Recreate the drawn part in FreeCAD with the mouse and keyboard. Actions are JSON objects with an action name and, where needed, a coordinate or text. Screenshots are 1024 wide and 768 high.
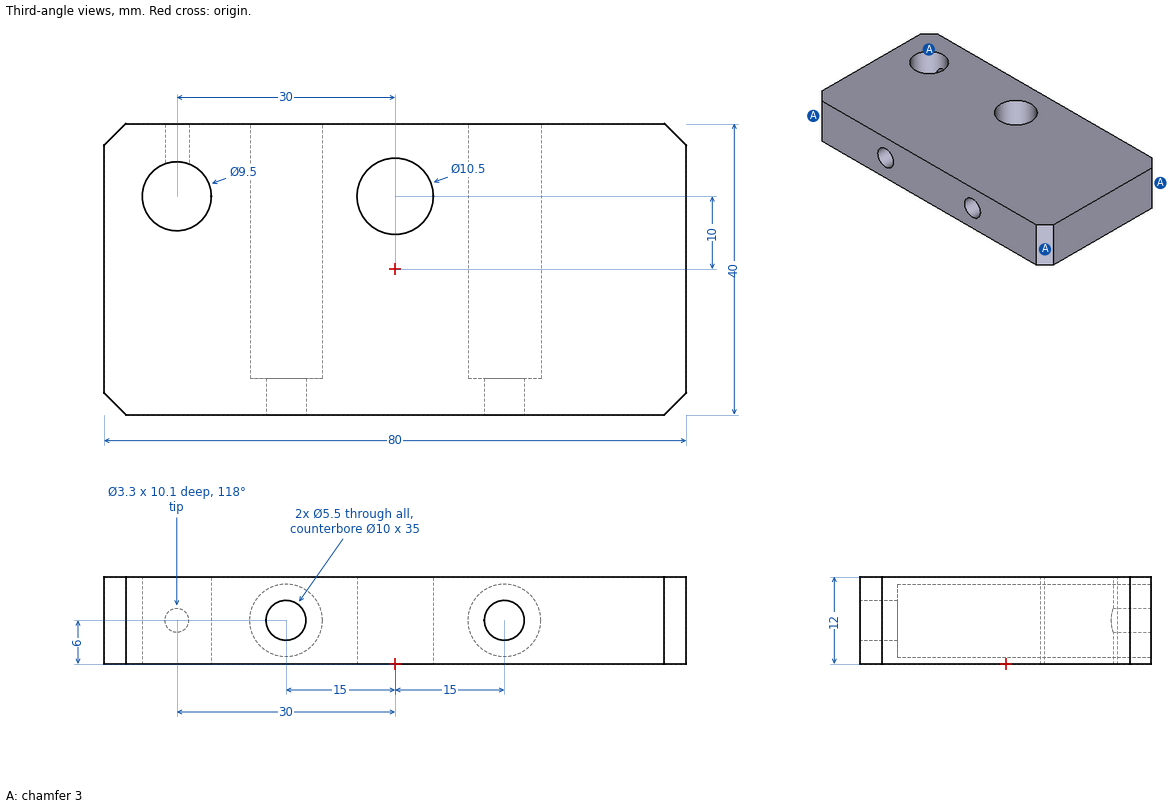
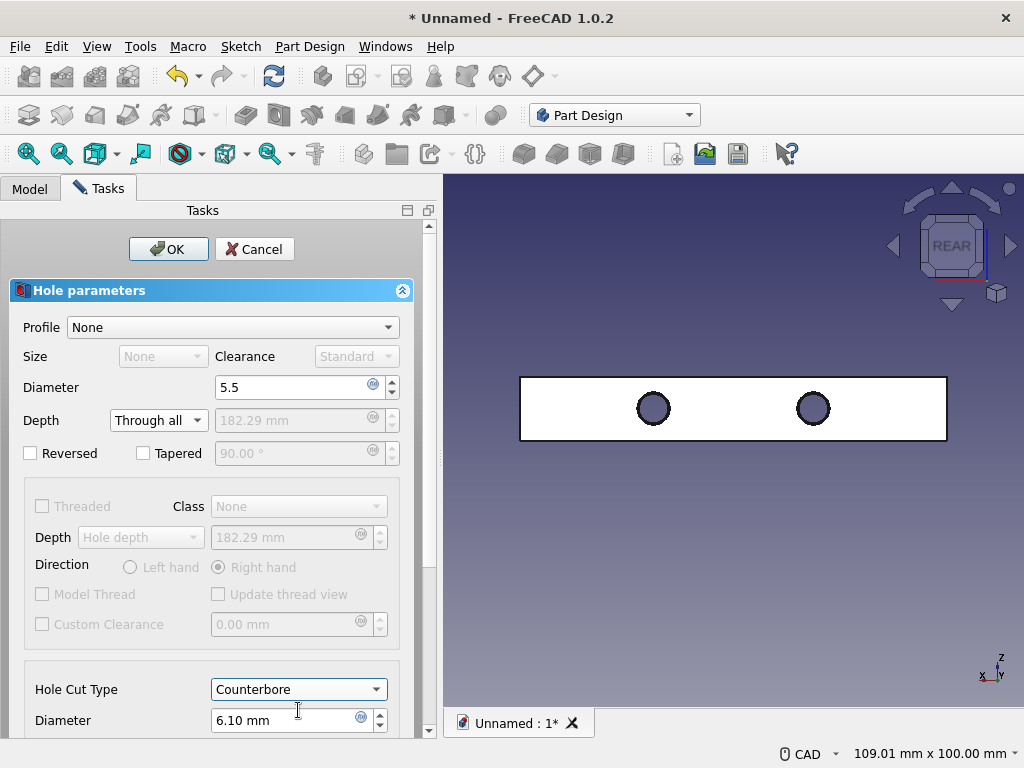
{"action": "triple_click", "coordinate": [292, 720]}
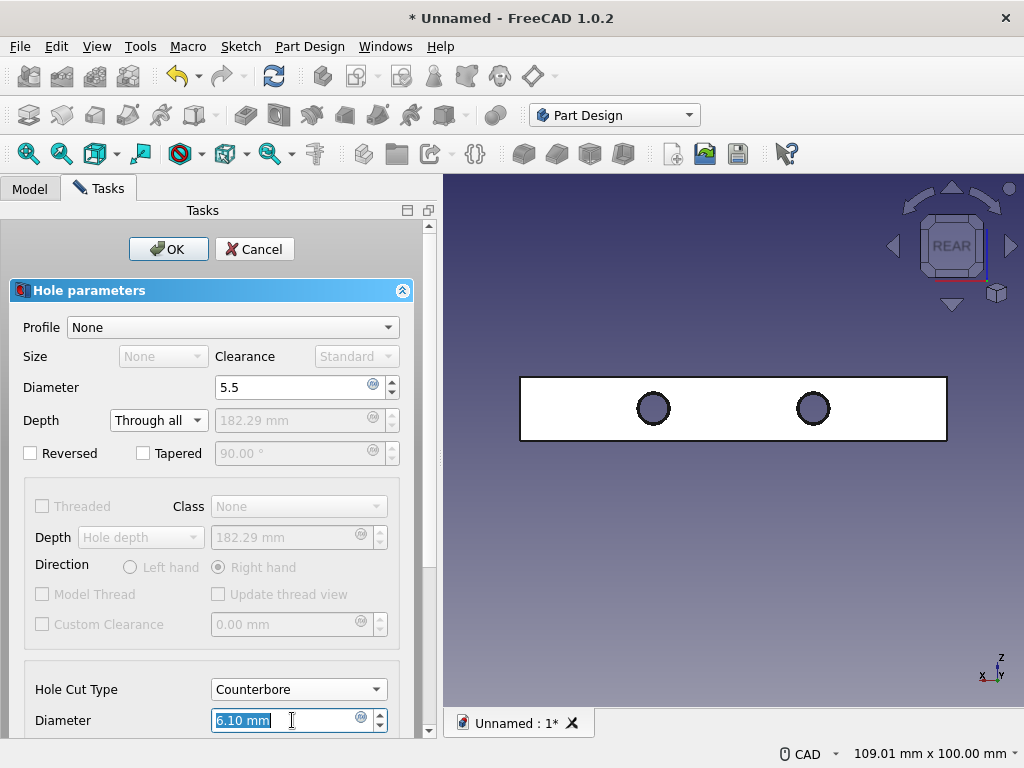
{"action": "type", "text": "10"}
{"action": "key", "text": "Tab"}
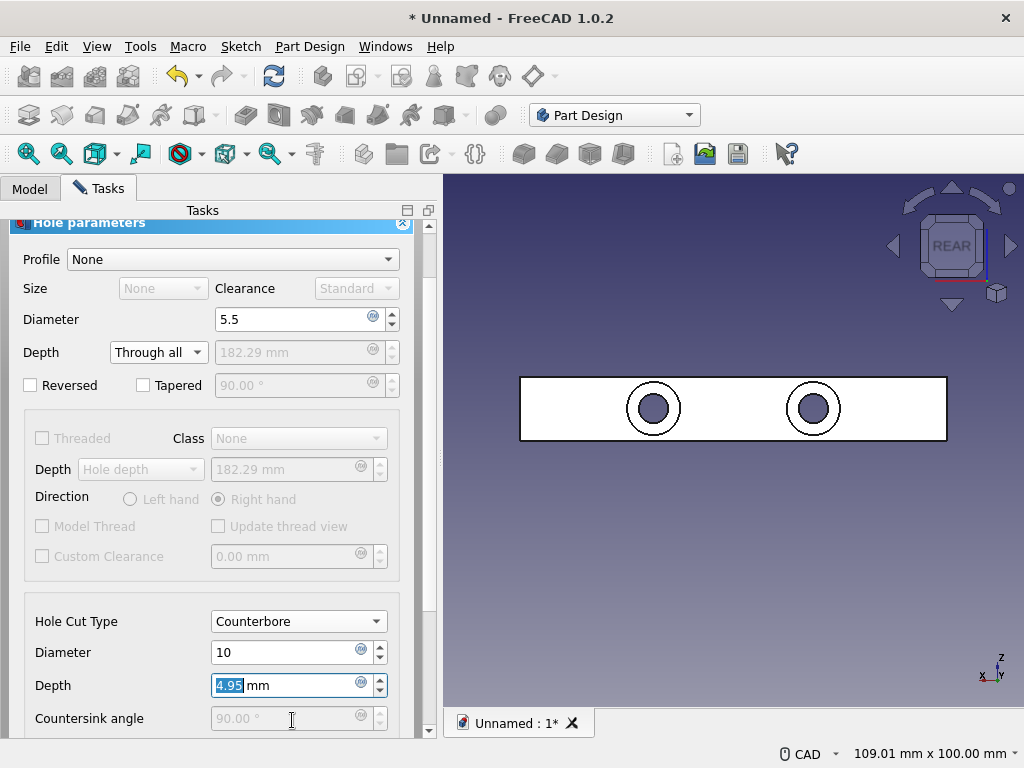
{"action": "type", "text": "35"}
{"action": "key", "text": "Tab"}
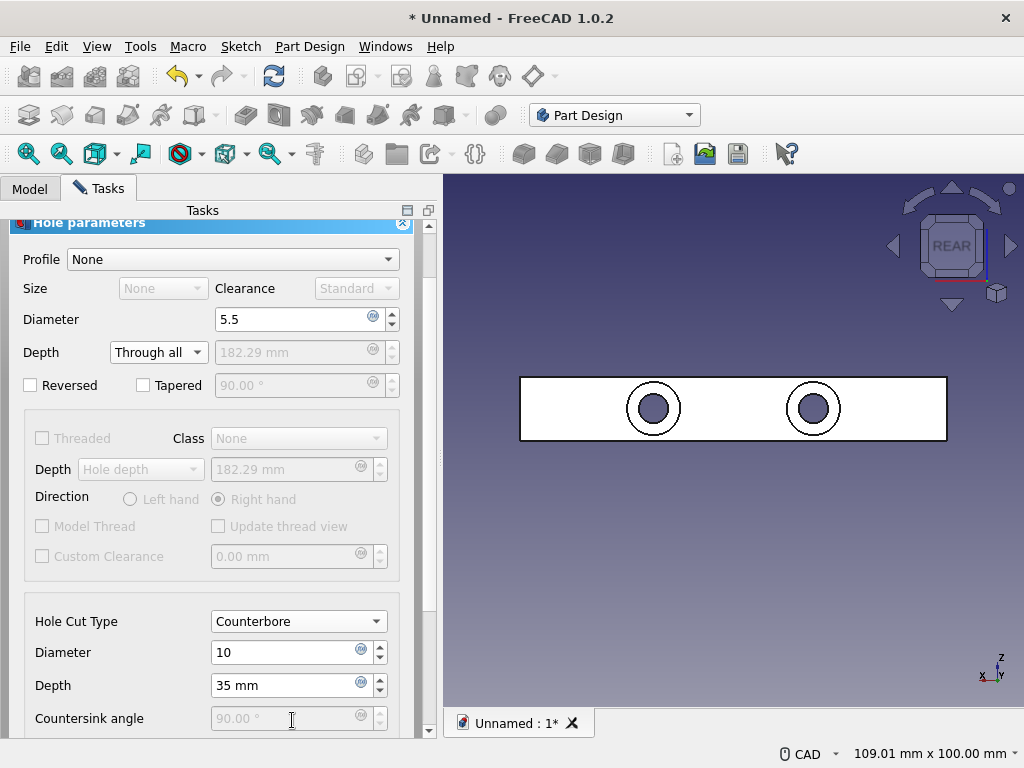
{"action": "scroll", "coordinate": [429, 479], "scroll_direction": "up", "scroll_amount": 2}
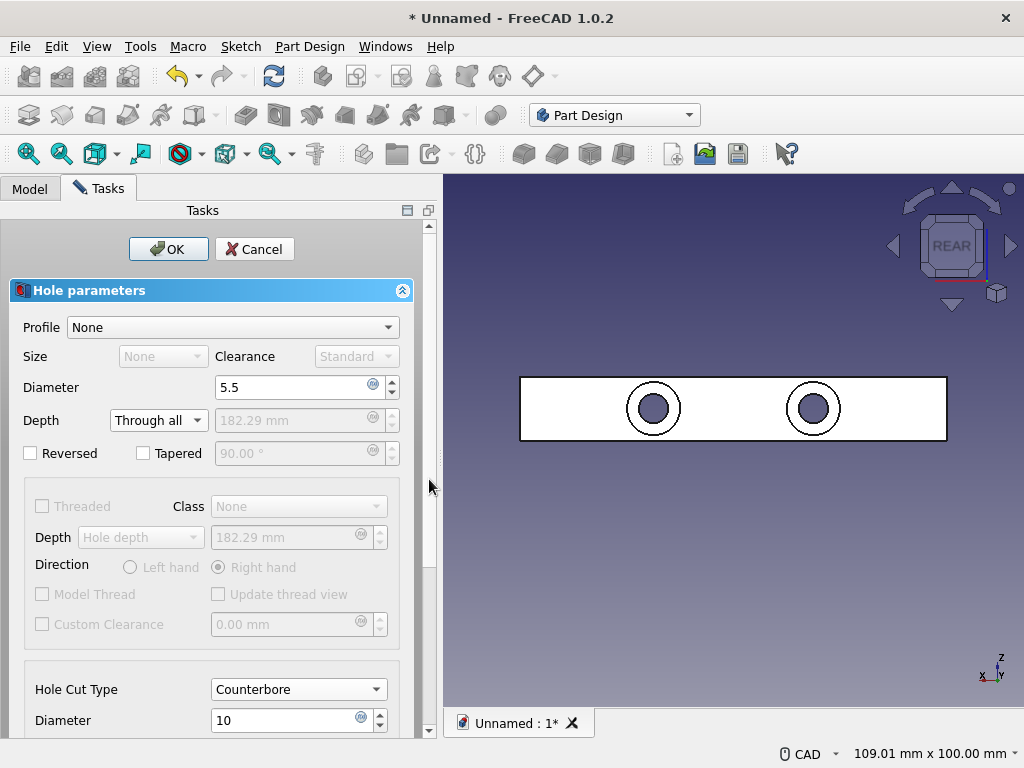
{"action": "left_click", "coordinate": [169, 249]}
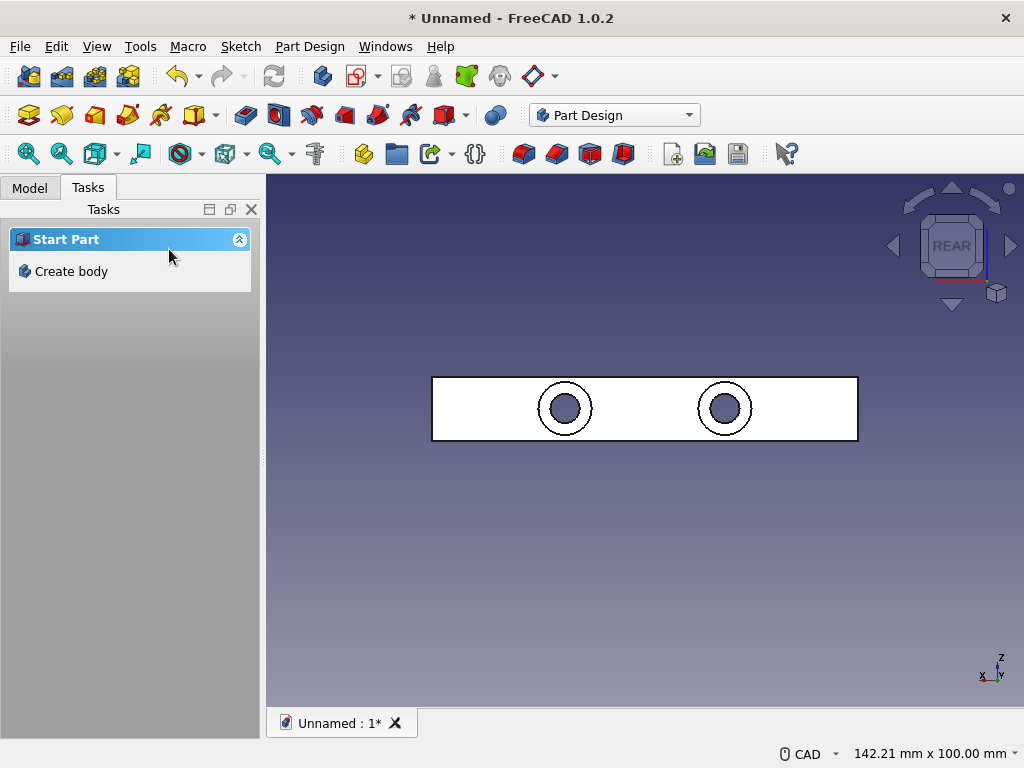
{"action": "left_click", "coordinate": [858, 408]}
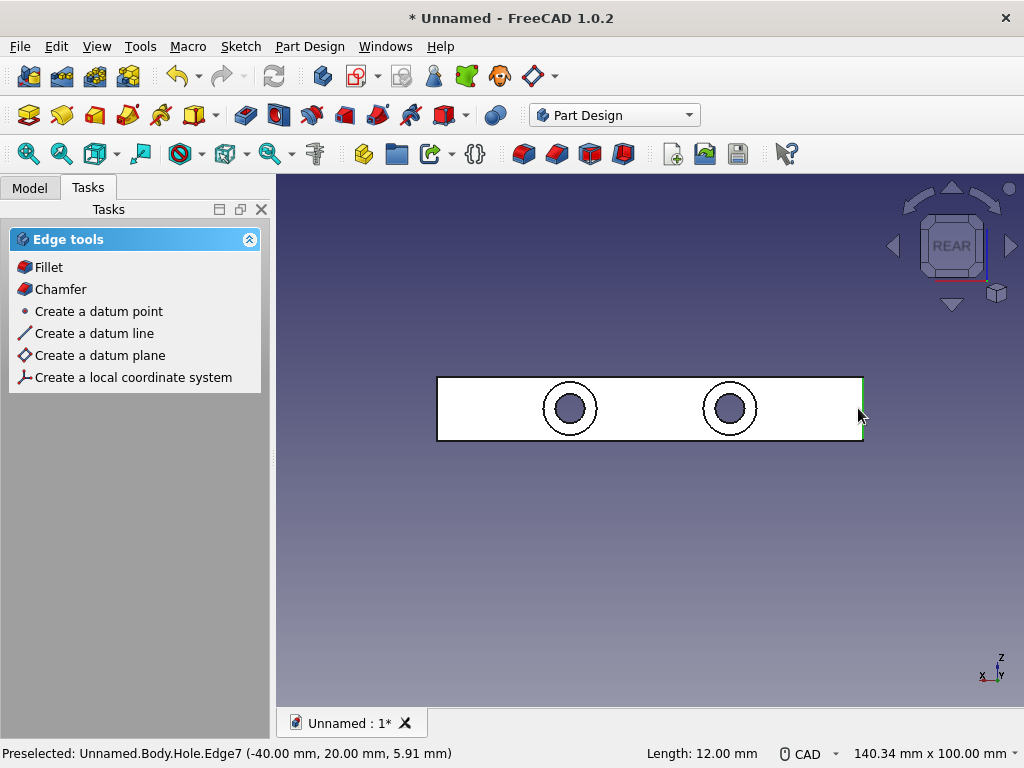
{"action": "key", "text": "0"}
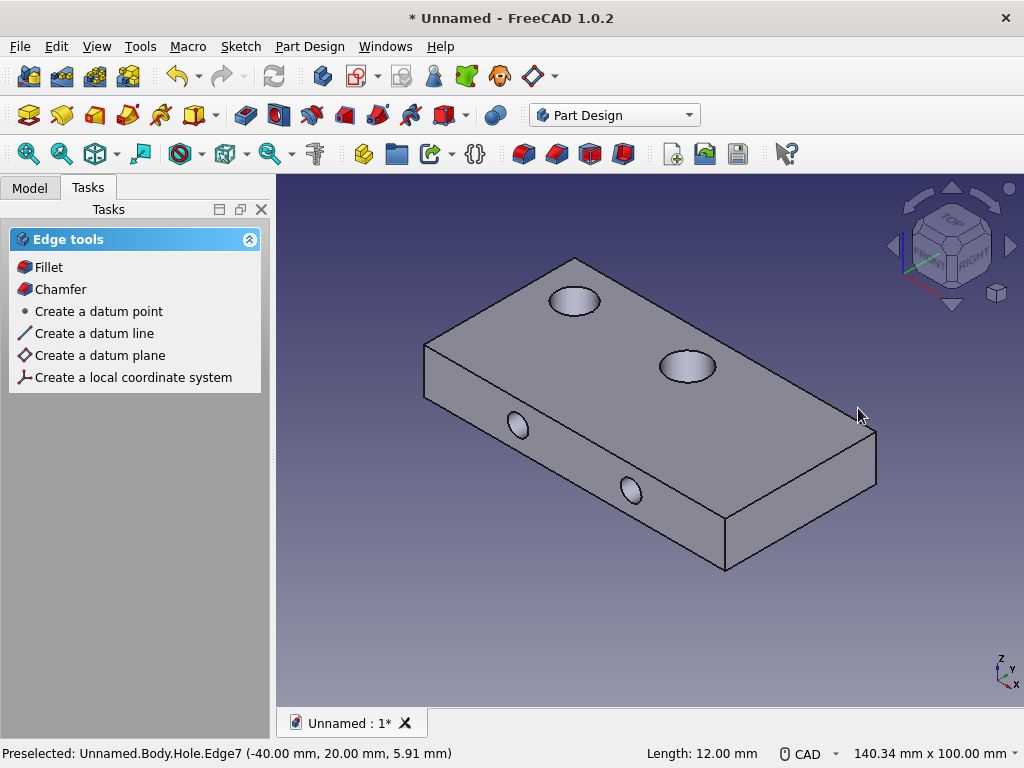
{"action": "left_click", "coordinate": [725, 544], "text": "ctrl"}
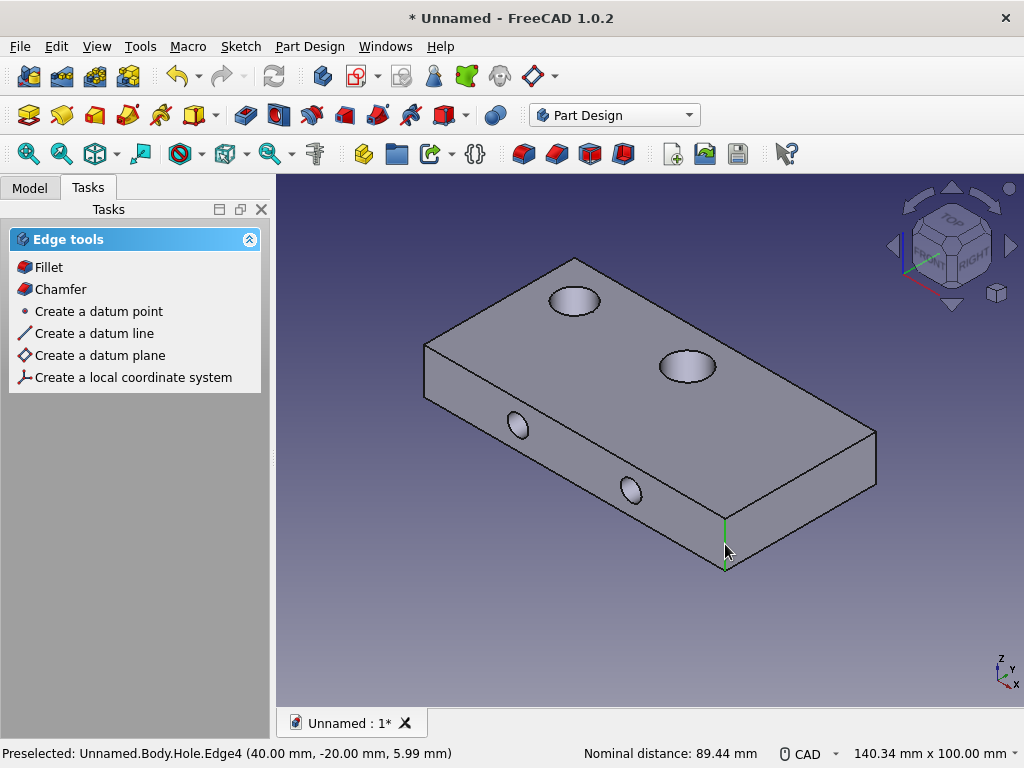
{"action": "key", "text": "2"}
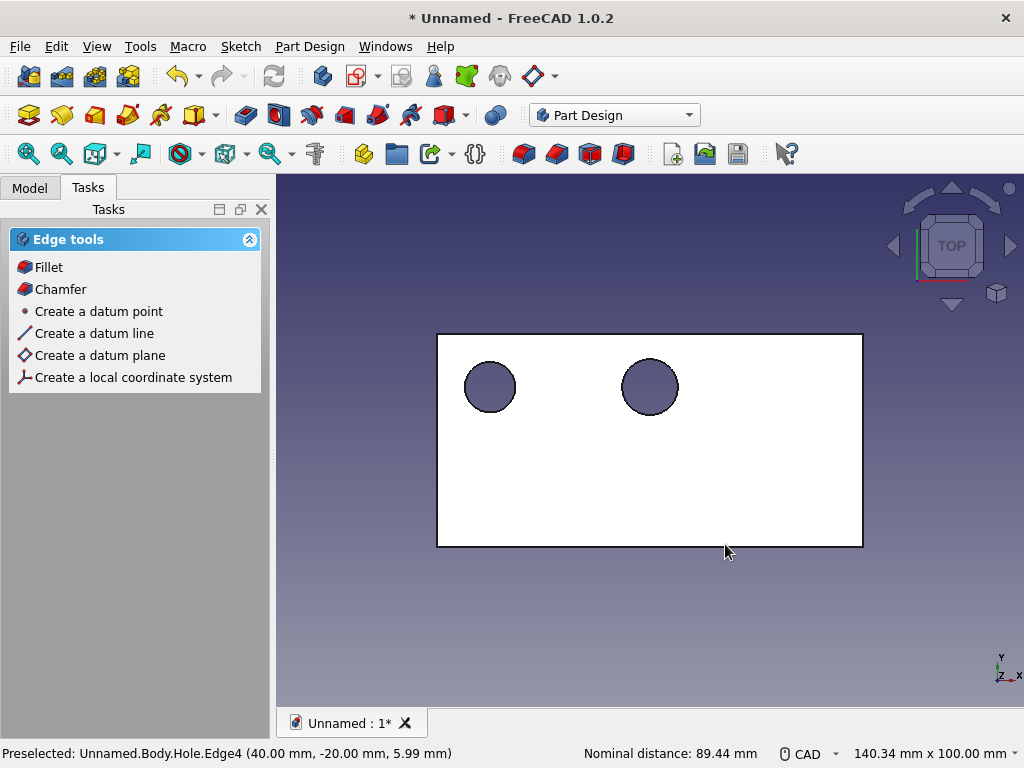
{"action": "key", "text": "1"}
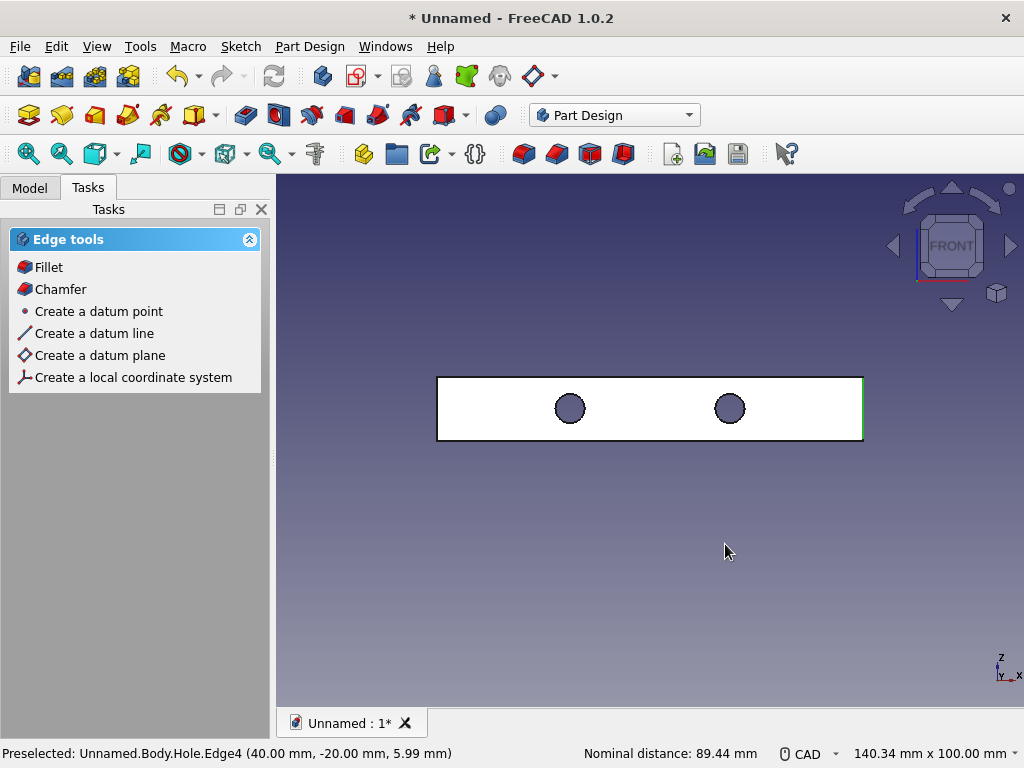
{"action": "left_click", "coordinate": [437, 408], "text": "ctrl"}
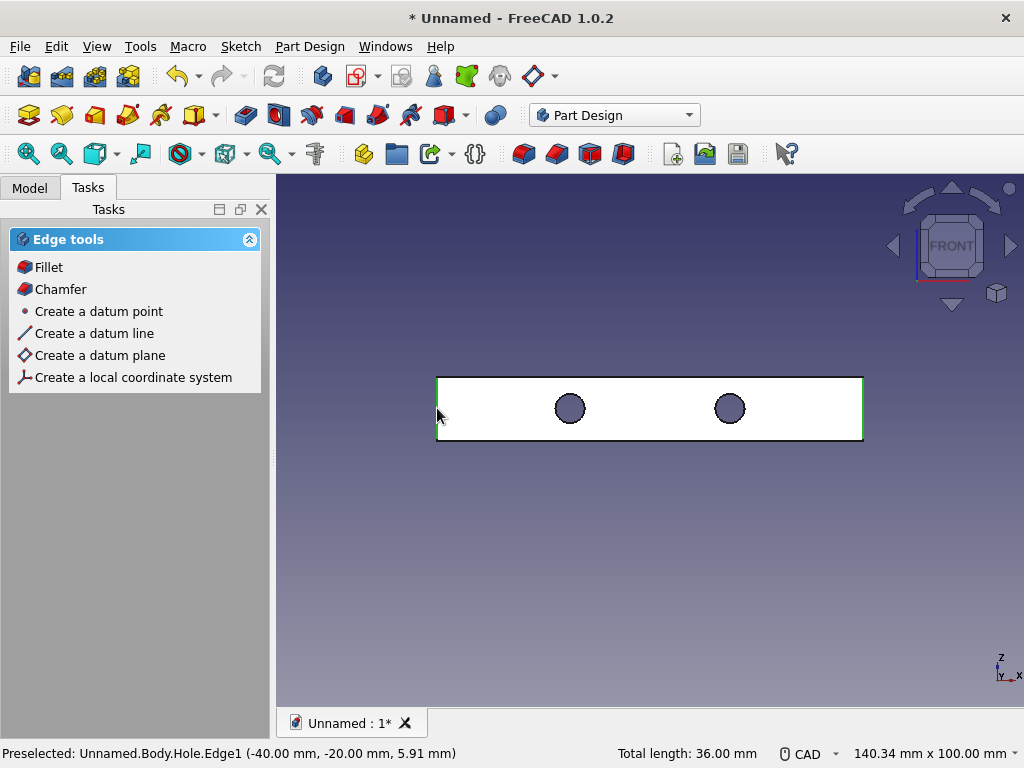
{"action": "key", "text": "3"}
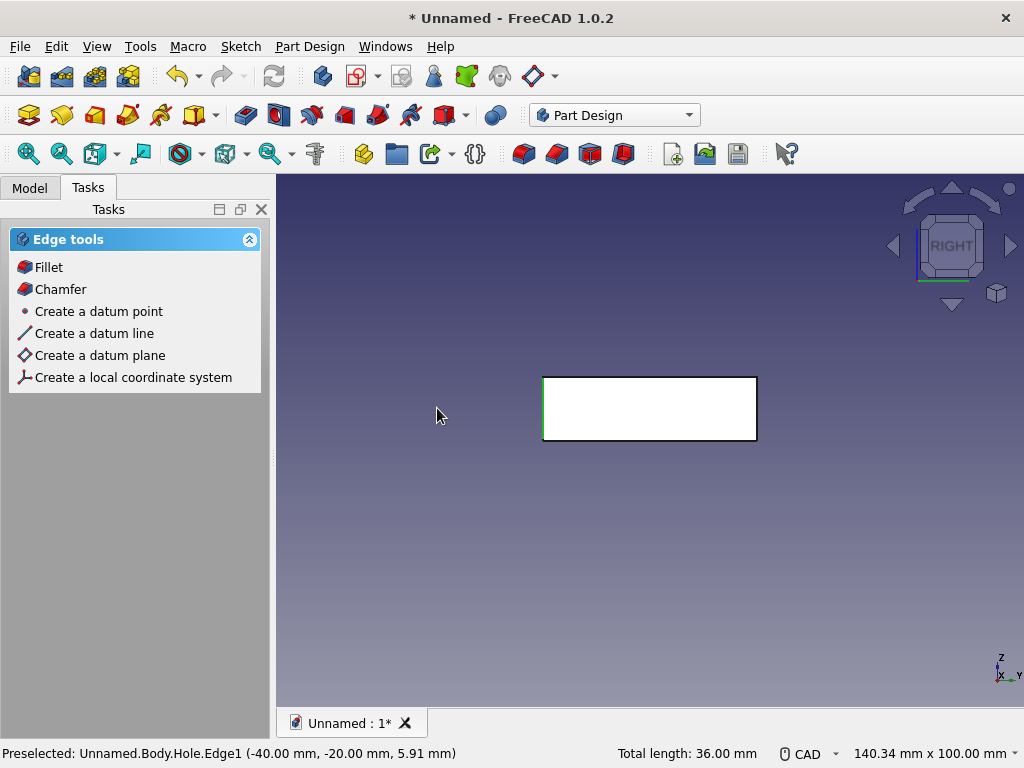
{"action": "key", "text": "v f"}